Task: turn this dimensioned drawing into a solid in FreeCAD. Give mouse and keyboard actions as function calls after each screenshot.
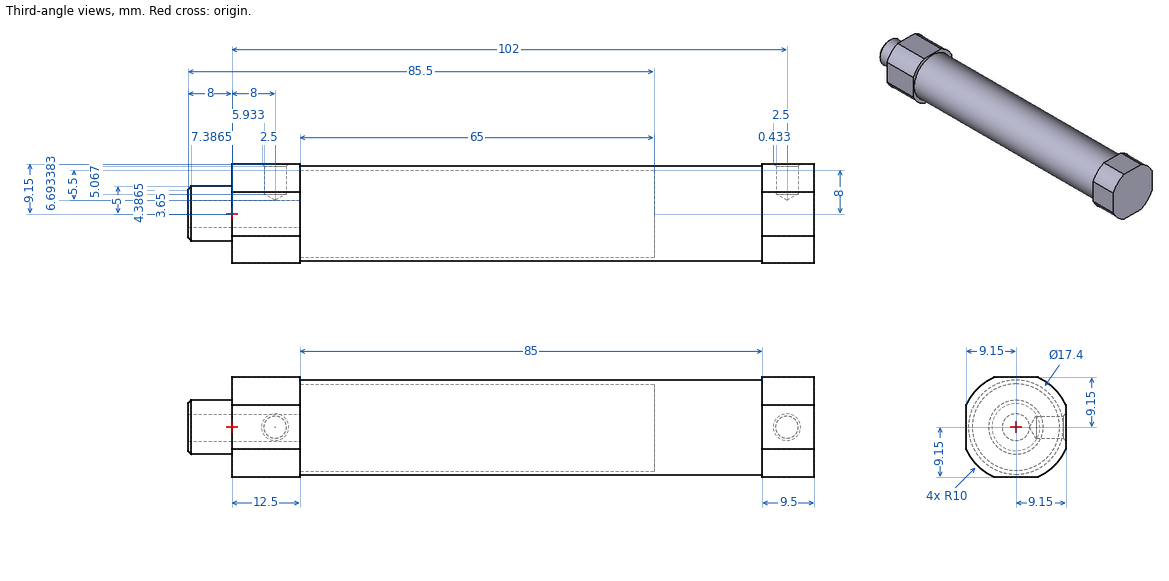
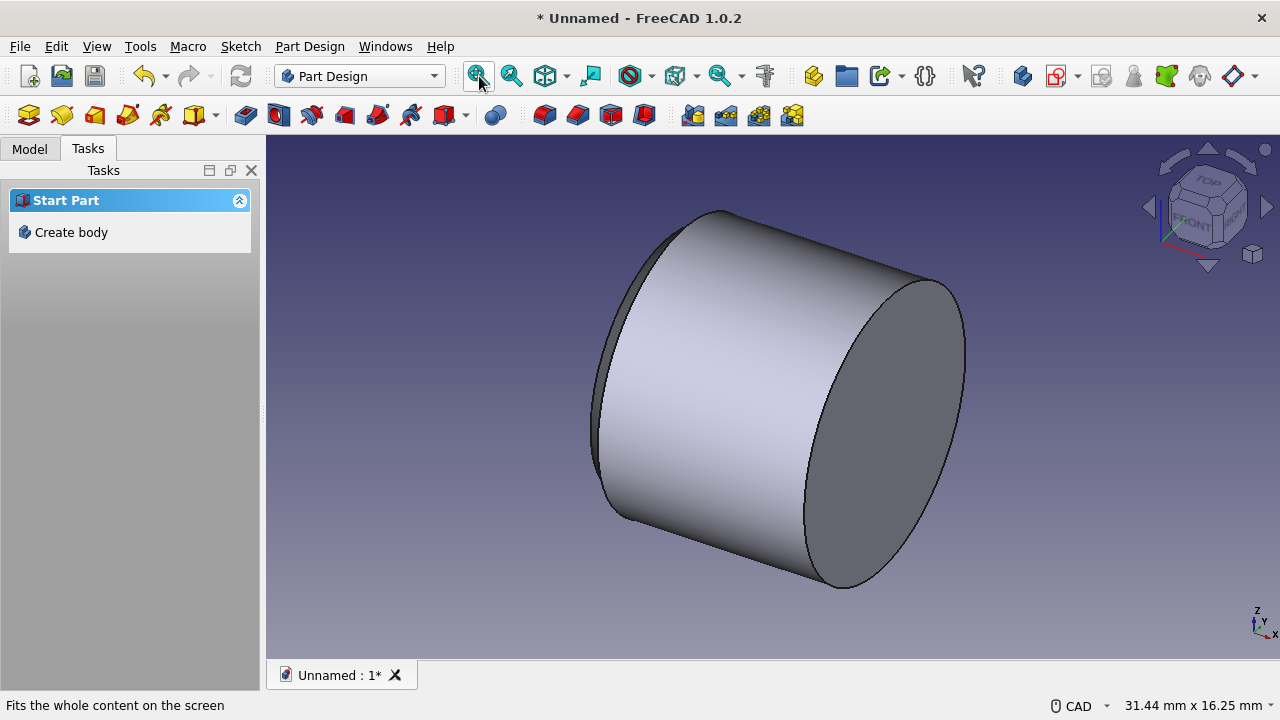
click(885, 433)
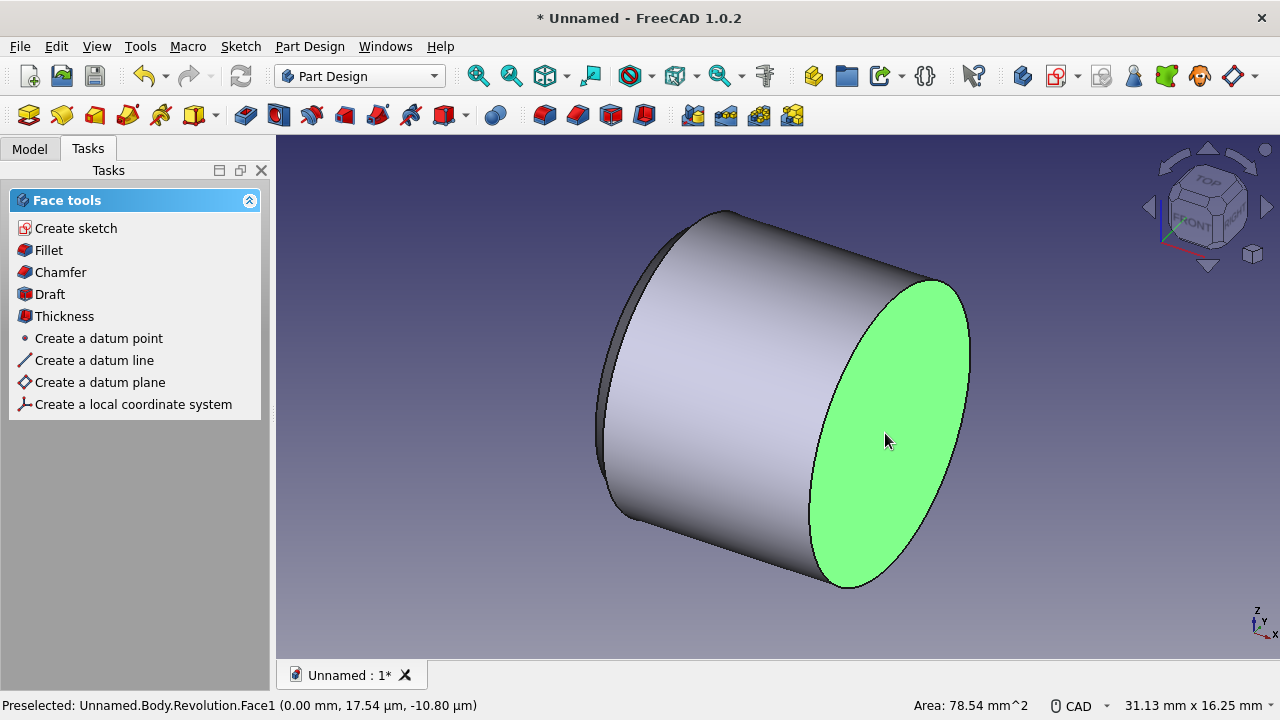
click(1056, 76)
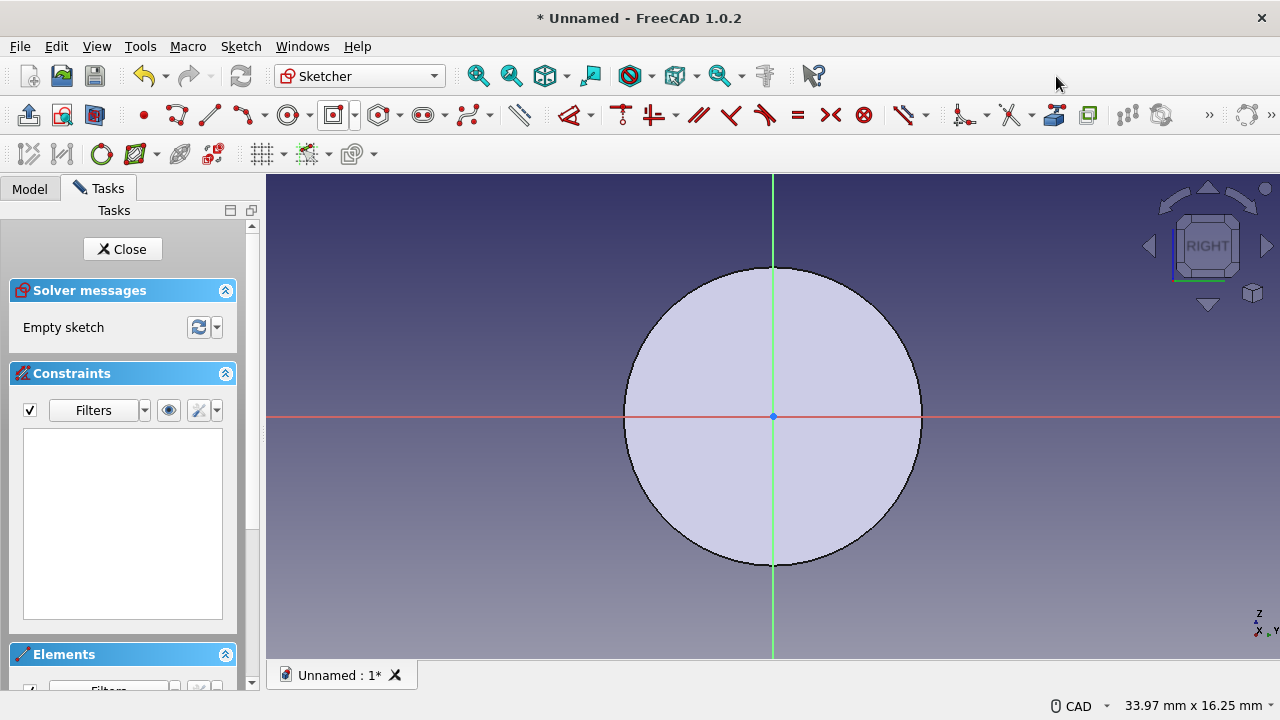
scroll(621, 416, down, 3)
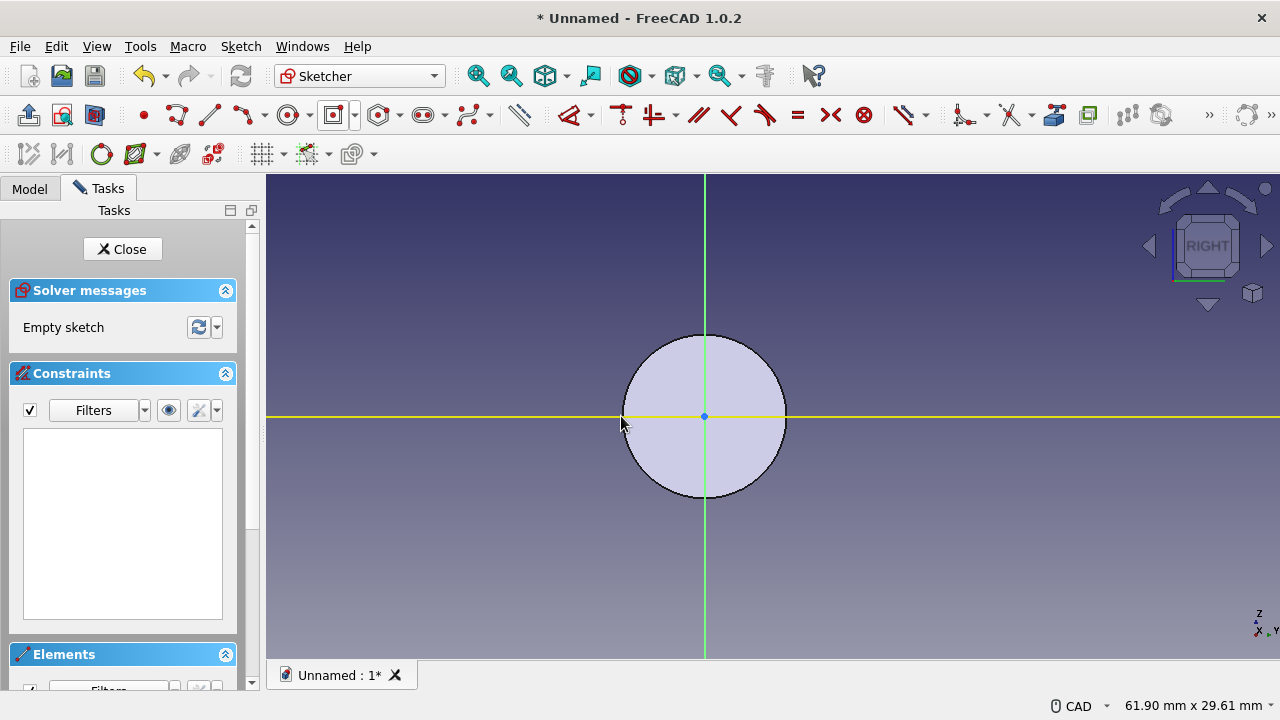
click(210, 116)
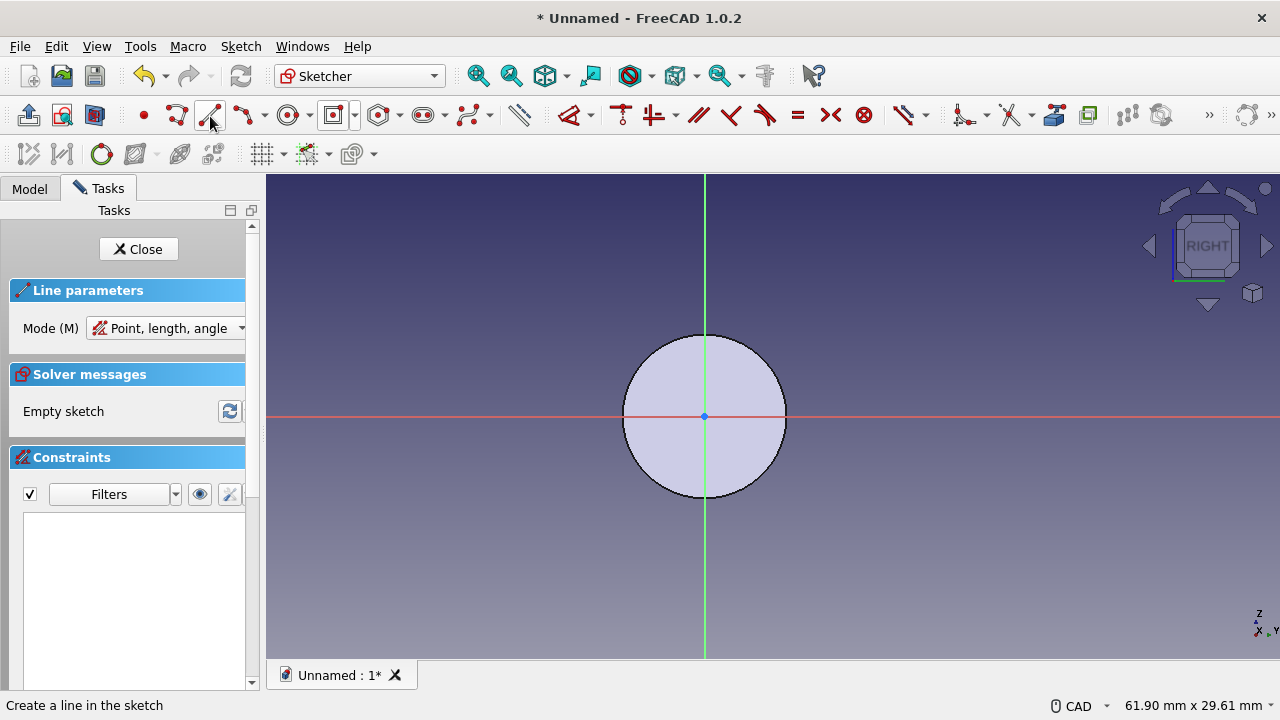
click(555, 350)
click(555, 483)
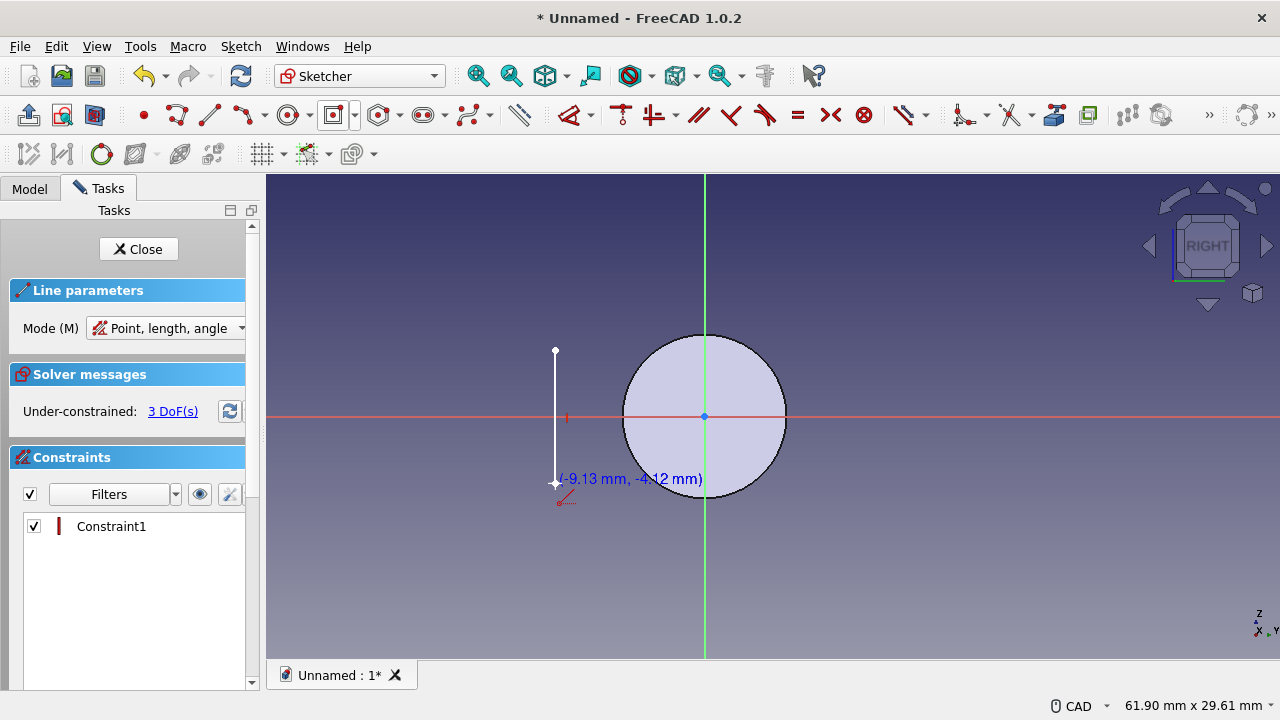
click(638, 566)
click(771, 566)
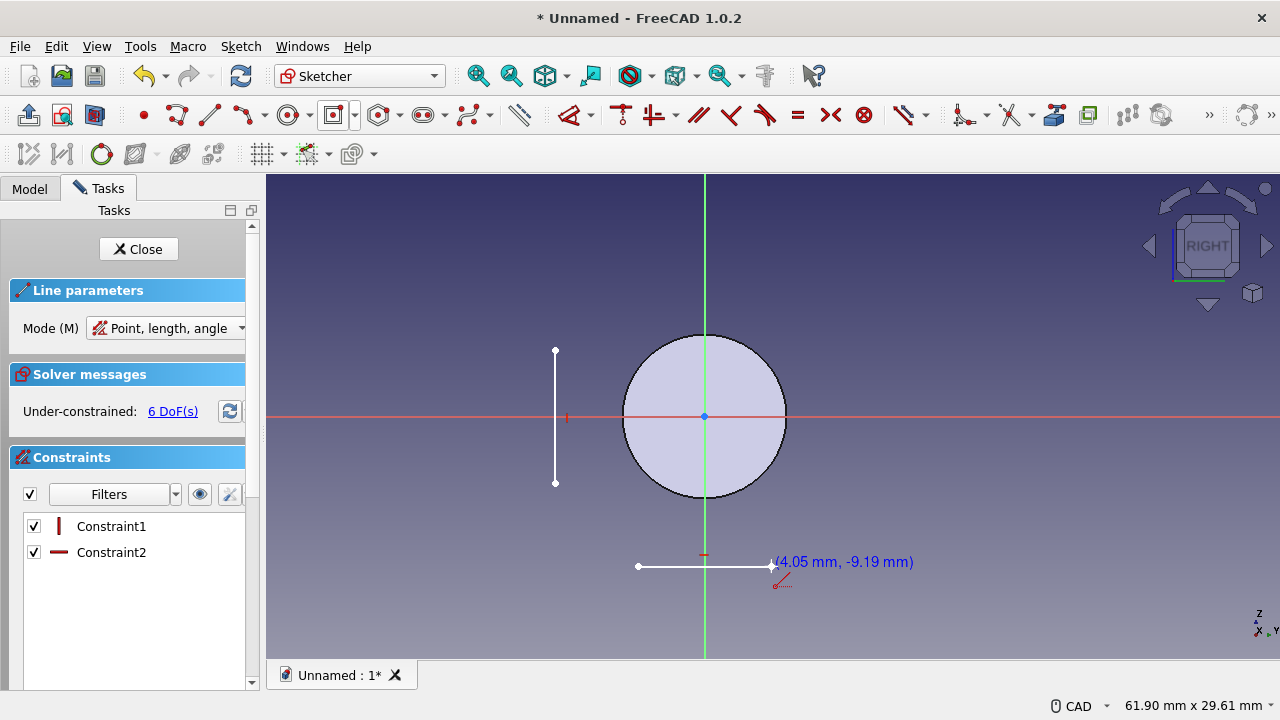
click(854, 483)
click(854, 350)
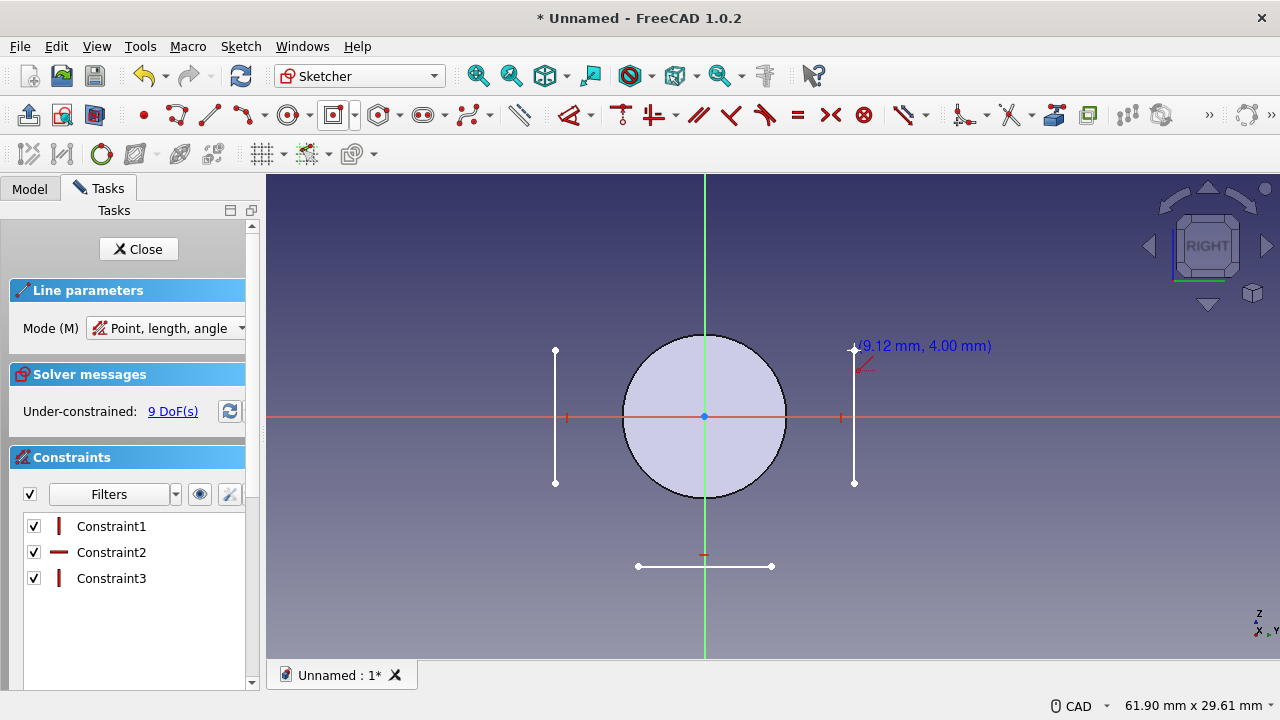
click(771, 267)
click(638, 267)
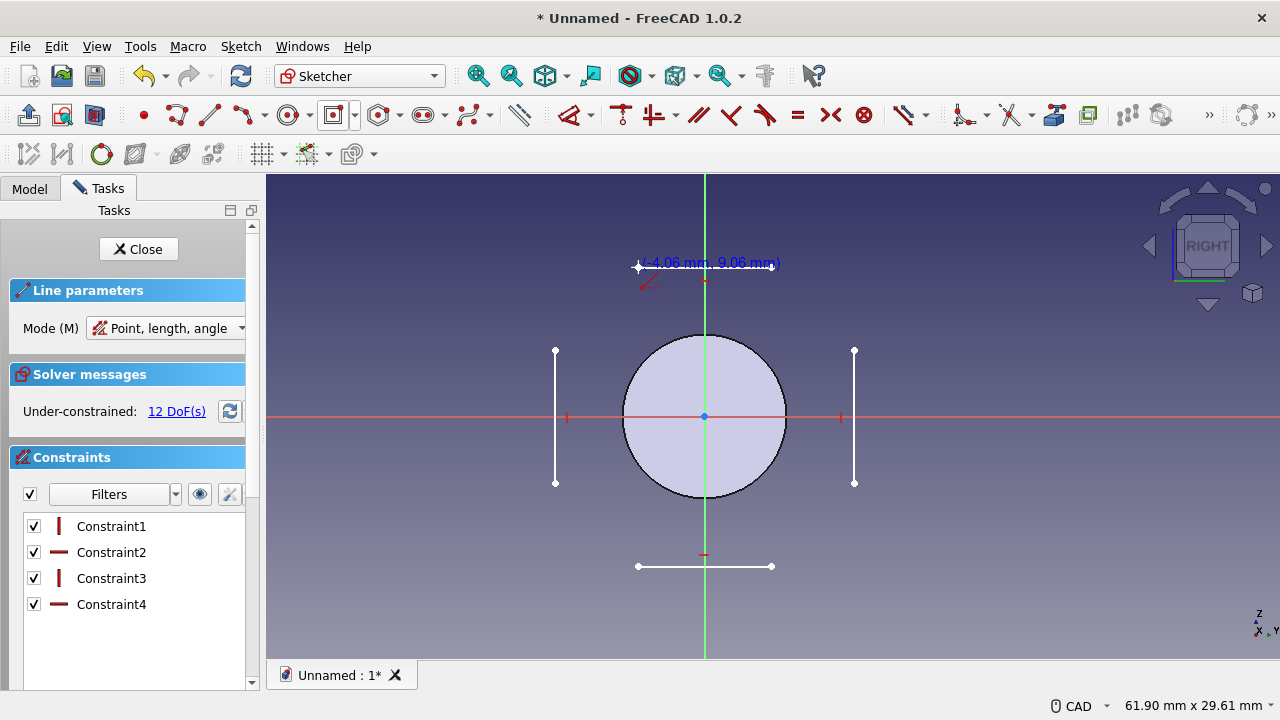
click(242, 116)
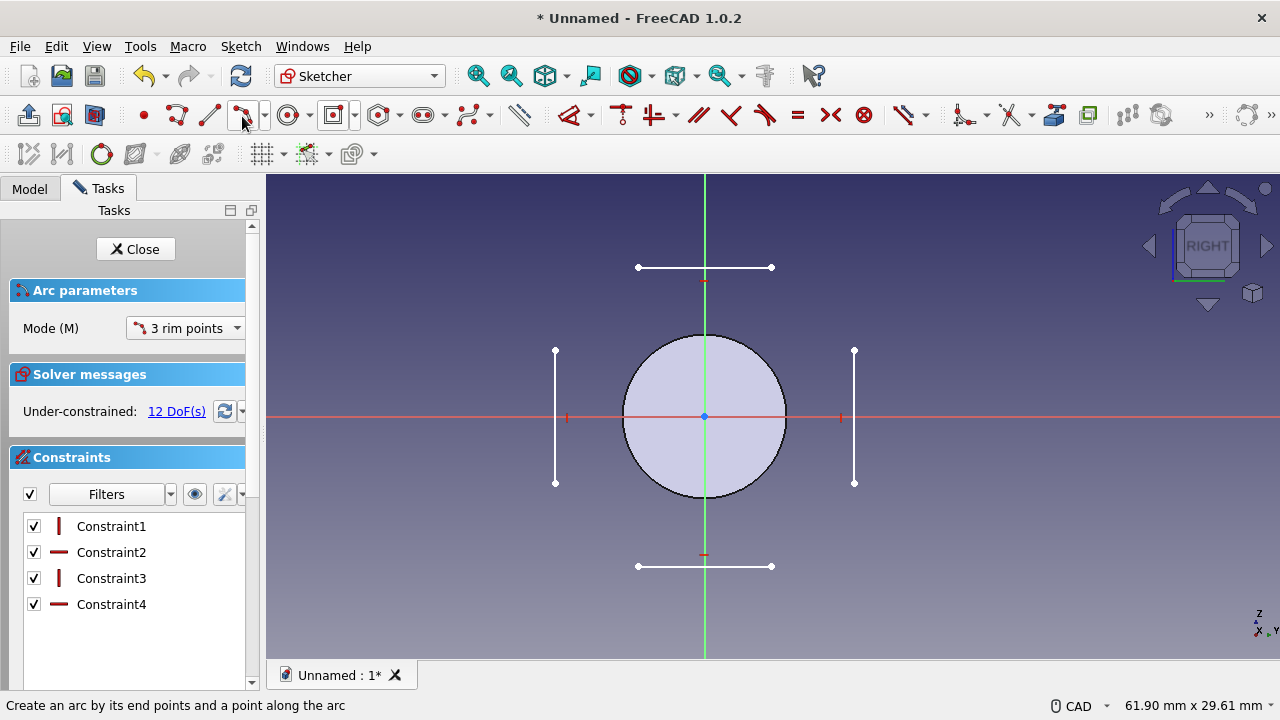
click(555, 484)
click(638, 567)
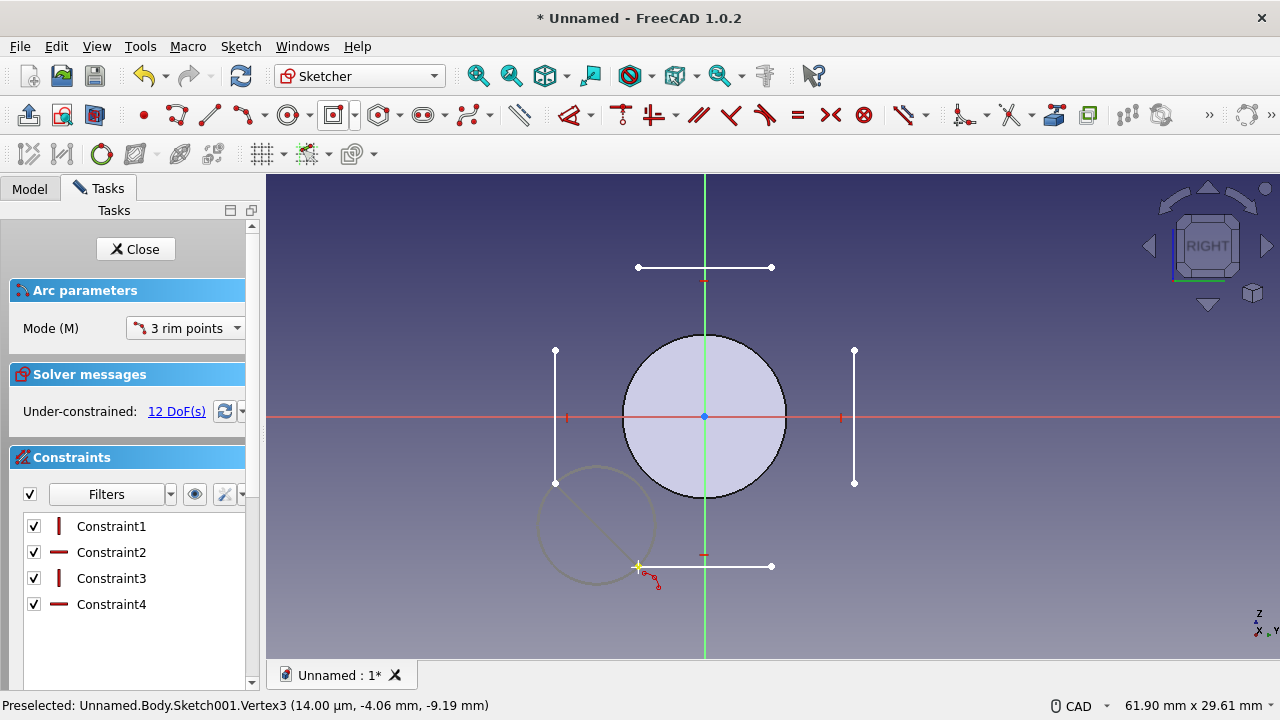
scroll(589, 532, up, 2)